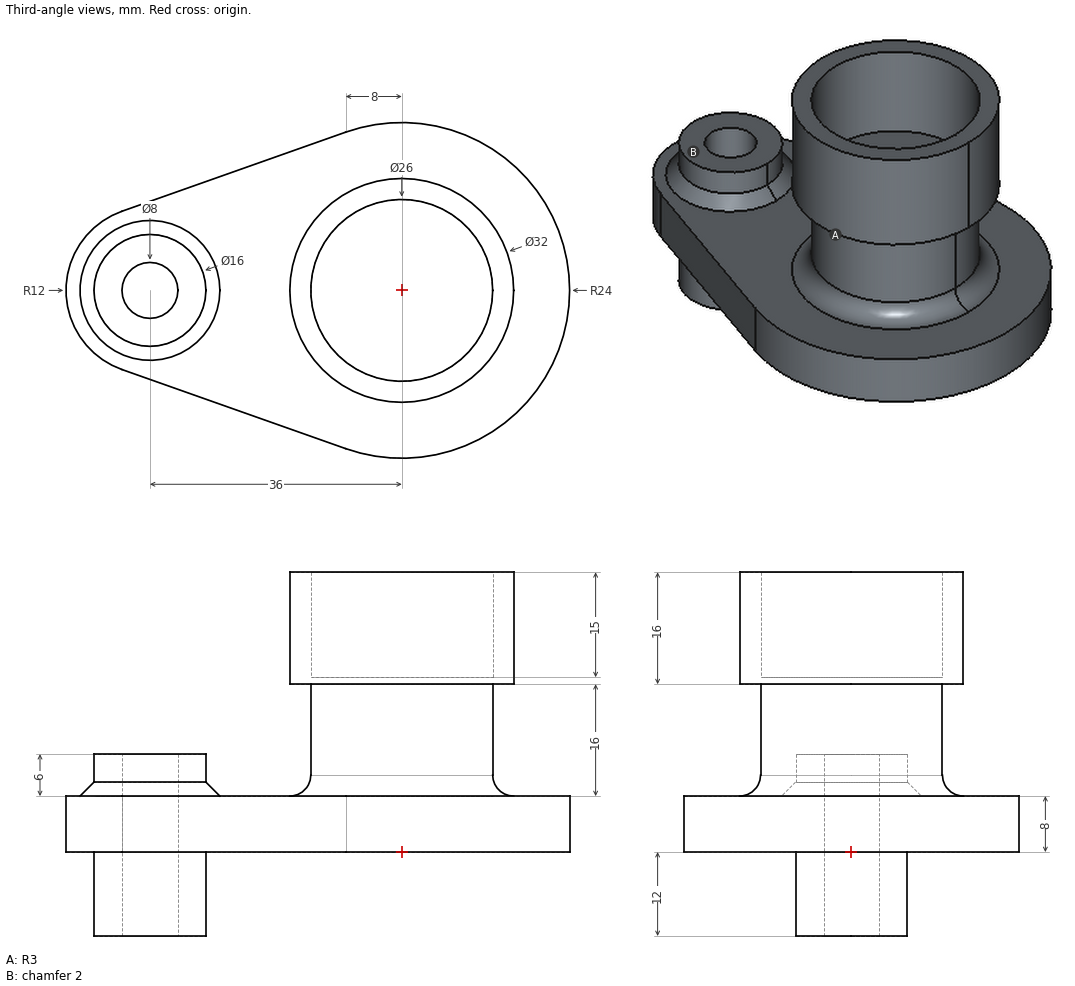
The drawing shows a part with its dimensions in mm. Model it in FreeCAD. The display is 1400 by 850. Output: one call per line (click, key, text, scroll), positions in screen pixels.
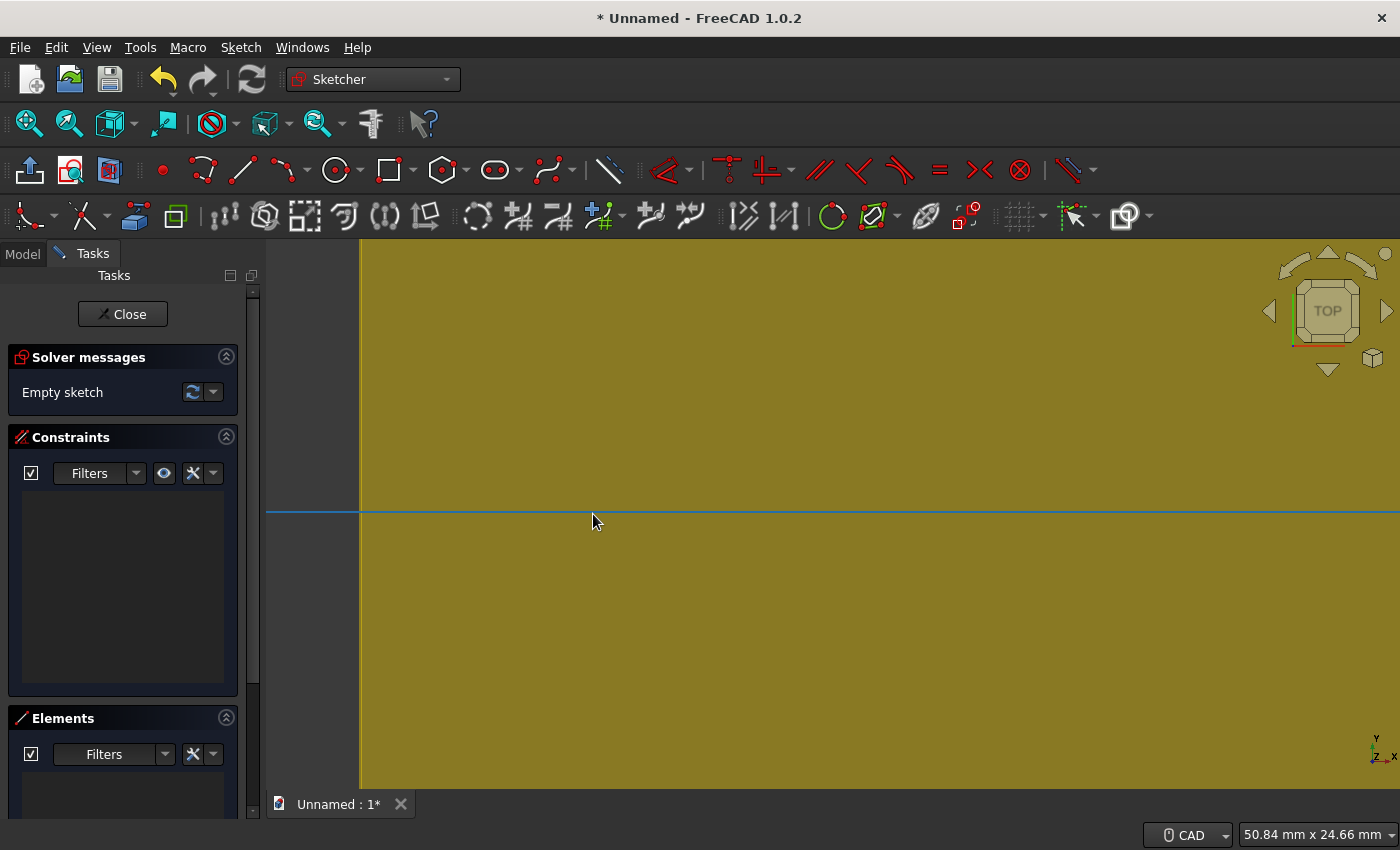
key(g)
key(c)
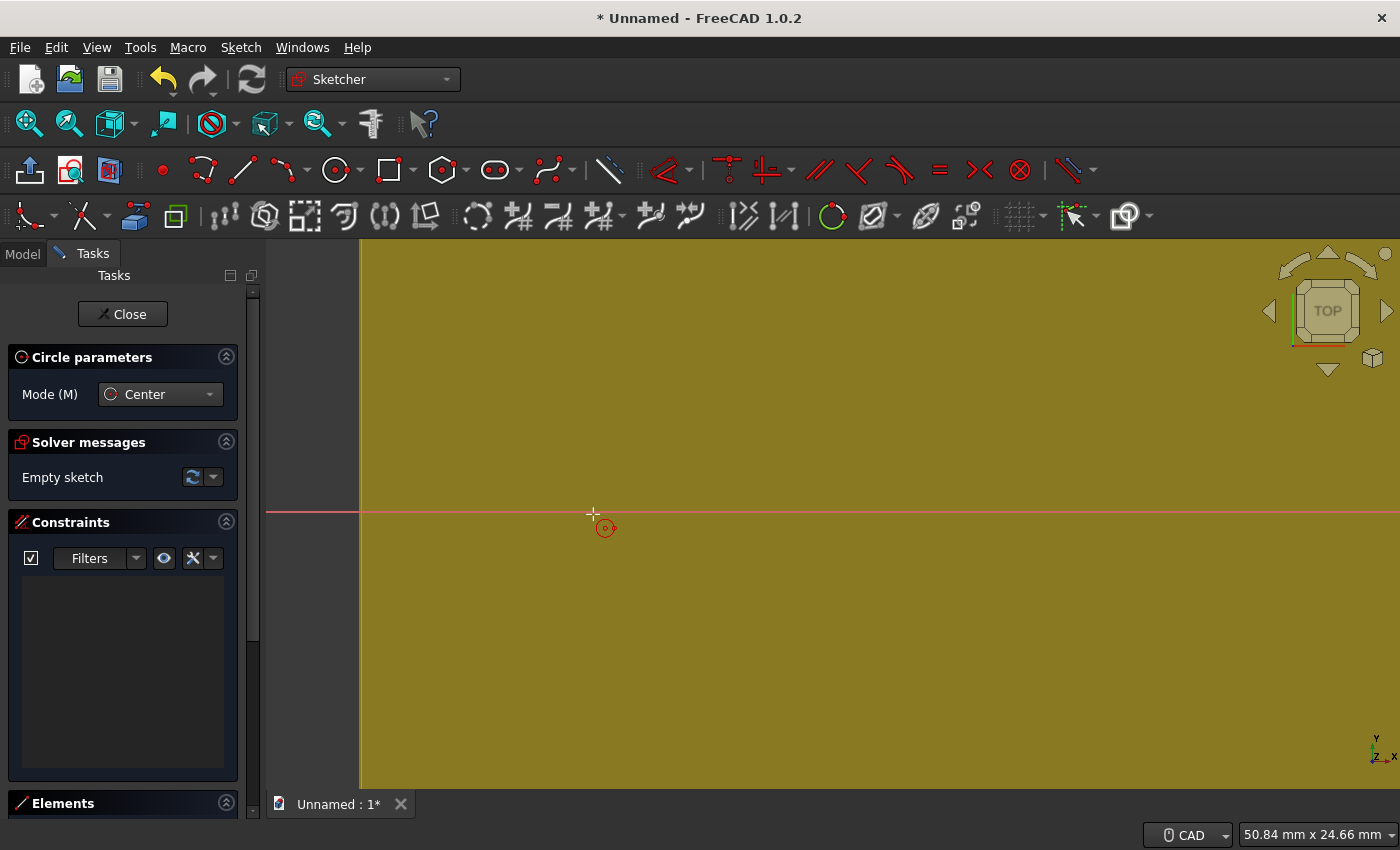
click(762, 512)
move(889, 386)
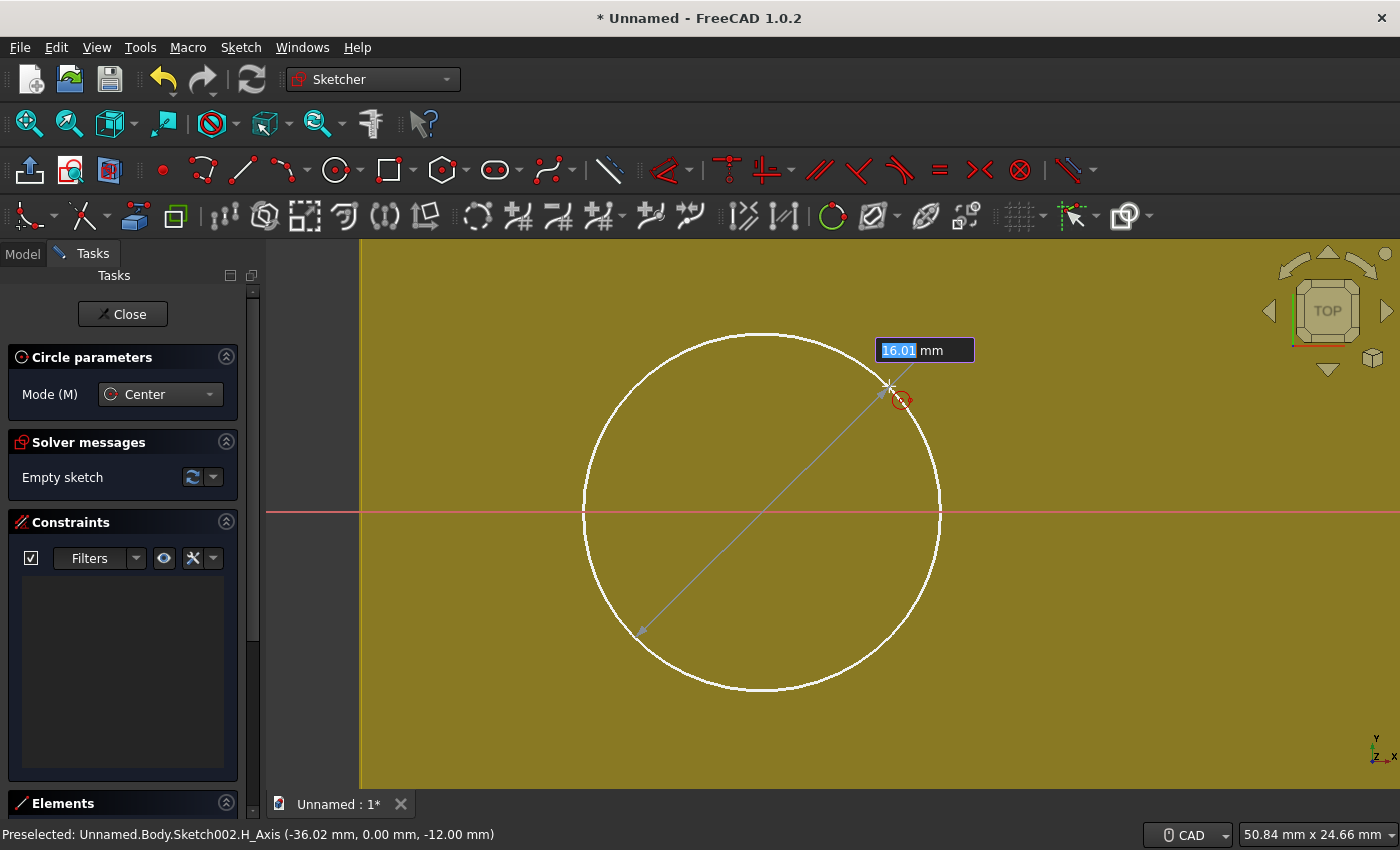
text(16)
key(Return)
key(Escape)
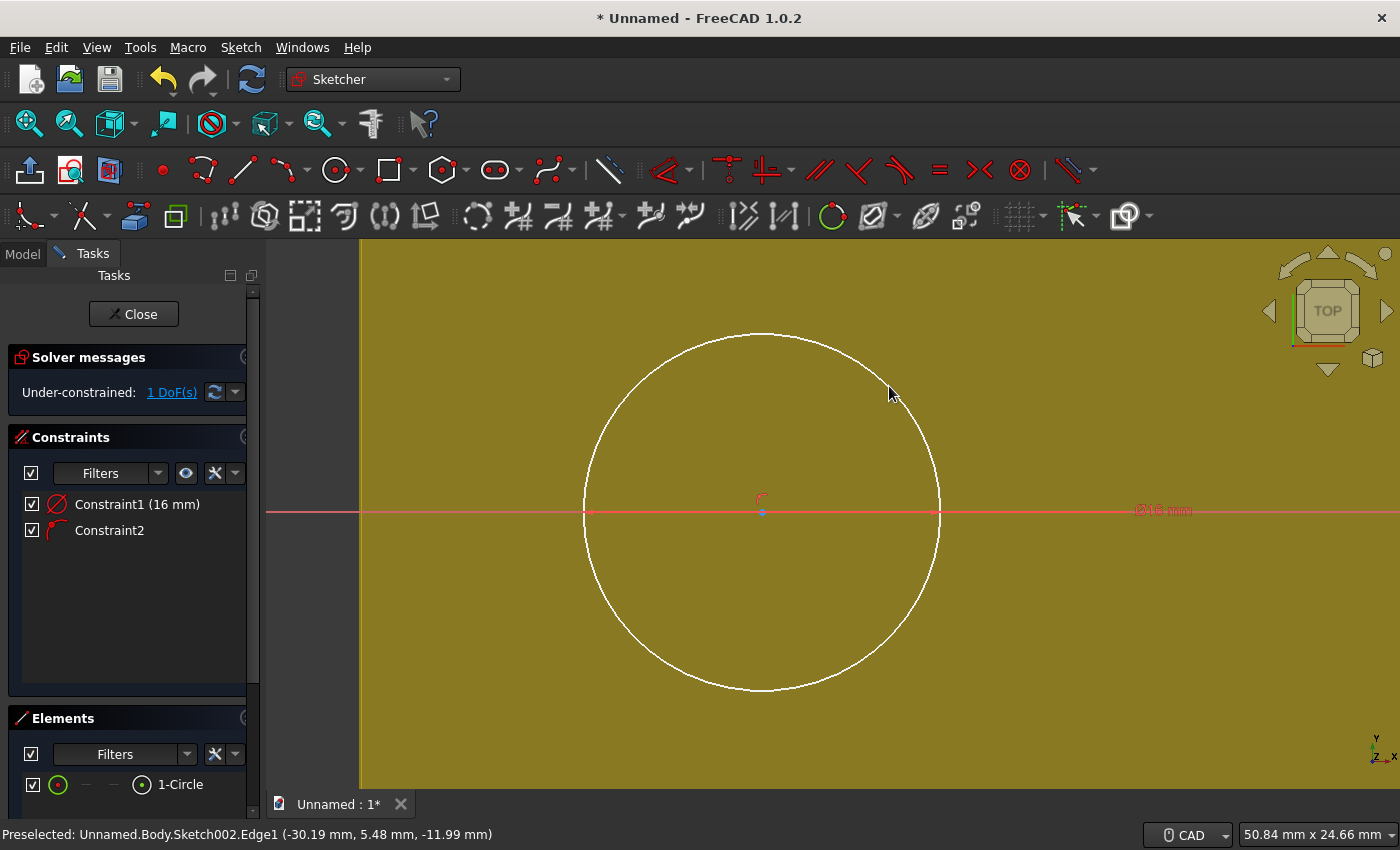
click(664, 170)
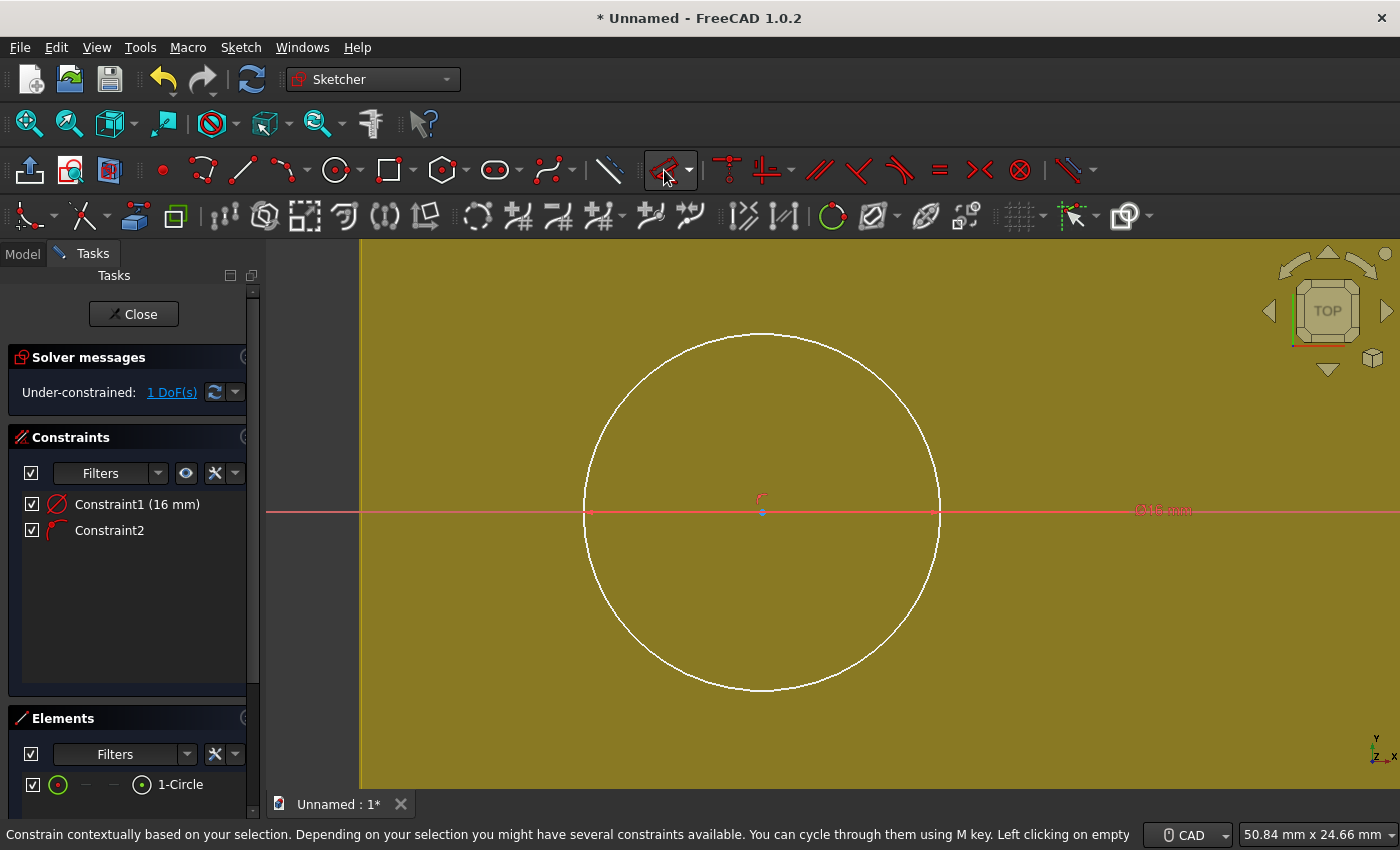
click(762, 512)
click(999, 546)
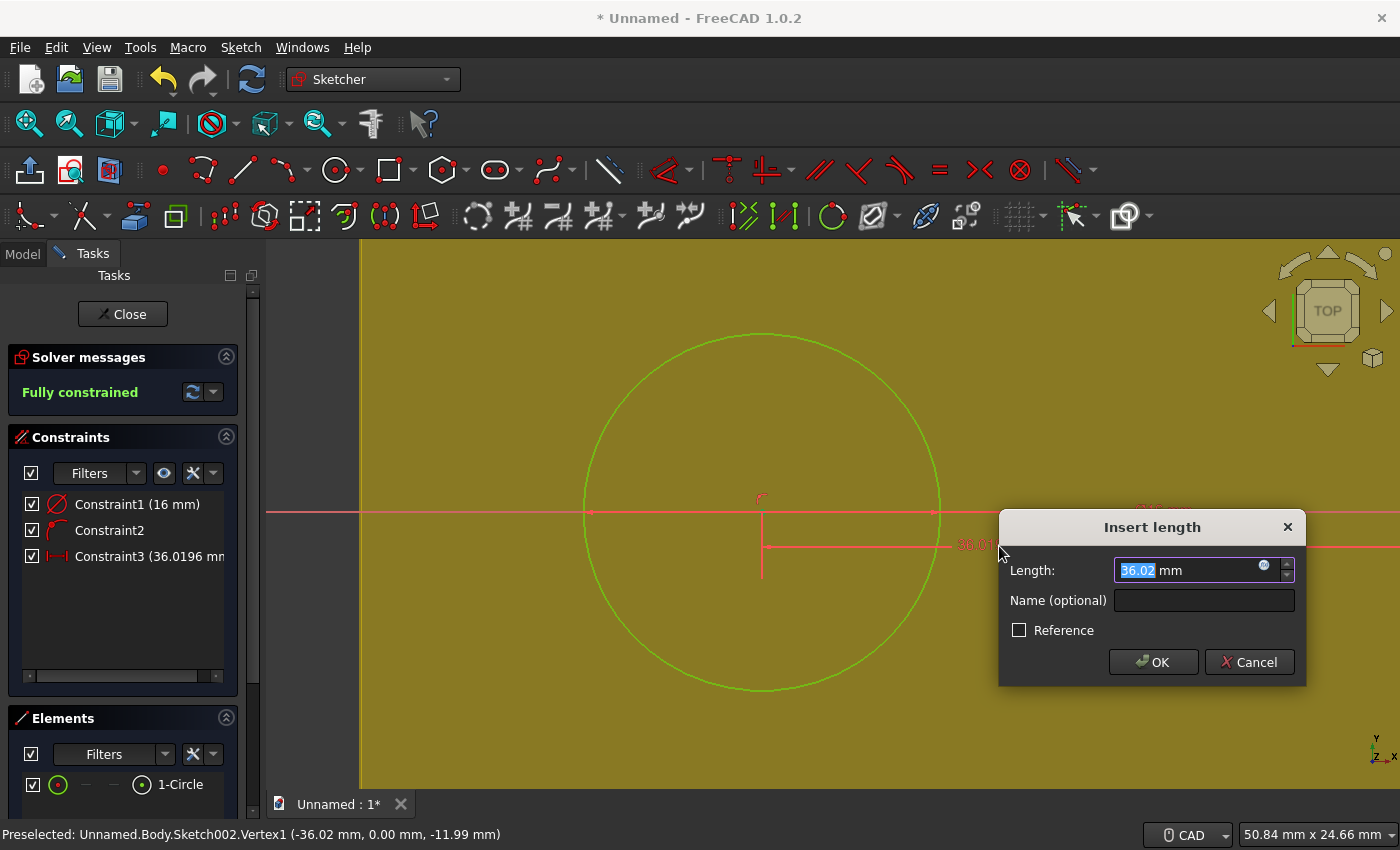
text(36)
key(Return)
key(Escape)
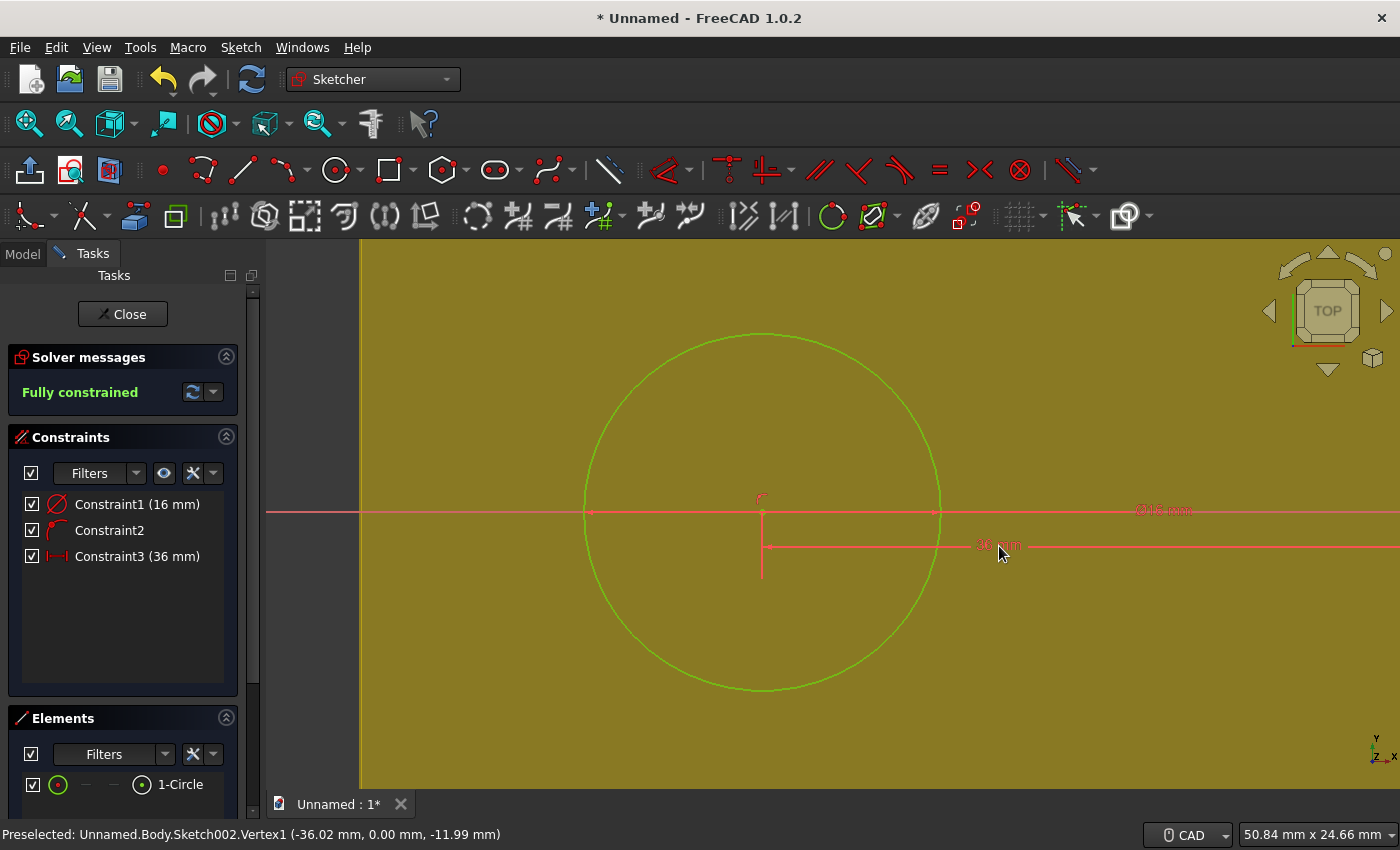
click(123, 314)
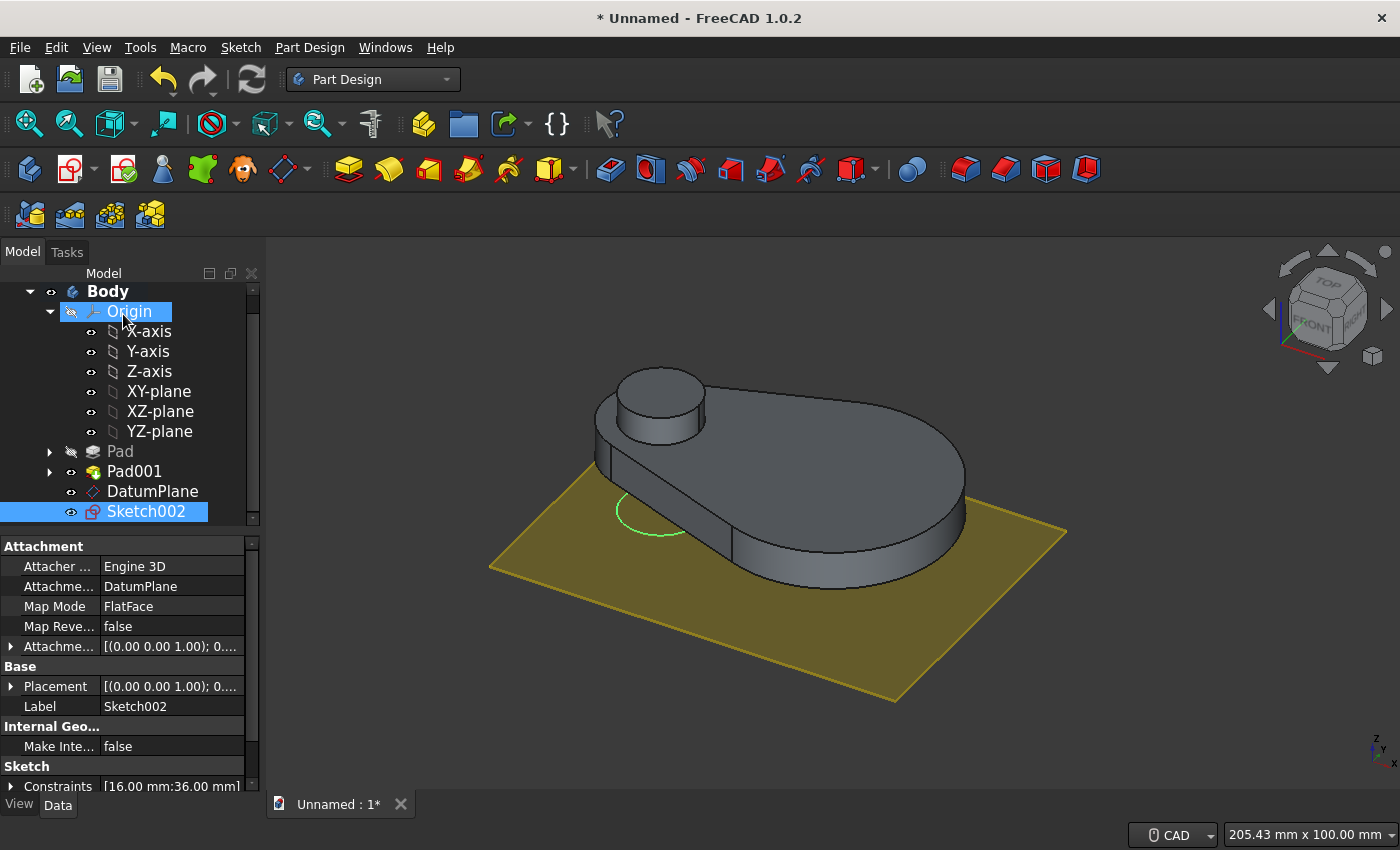
click(350, 170)